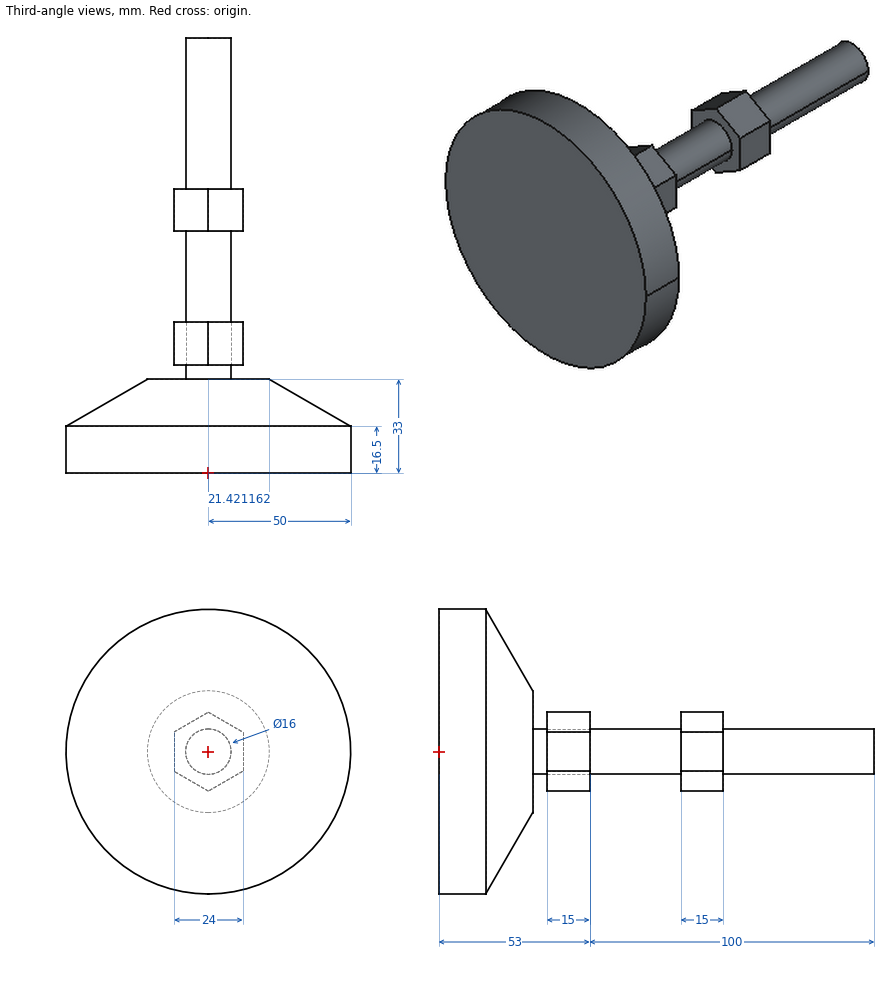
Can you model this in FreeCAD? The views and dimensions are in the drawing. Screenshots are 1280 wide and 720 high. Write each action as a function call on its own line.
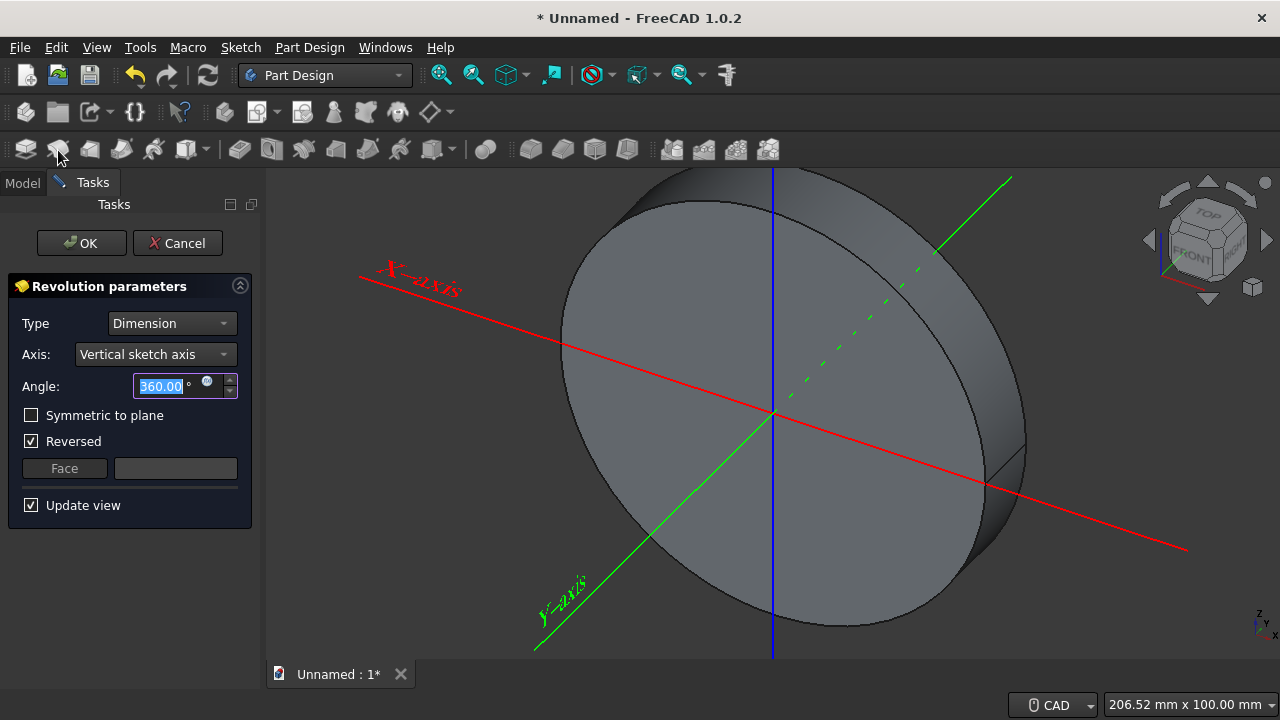
click(82, 243)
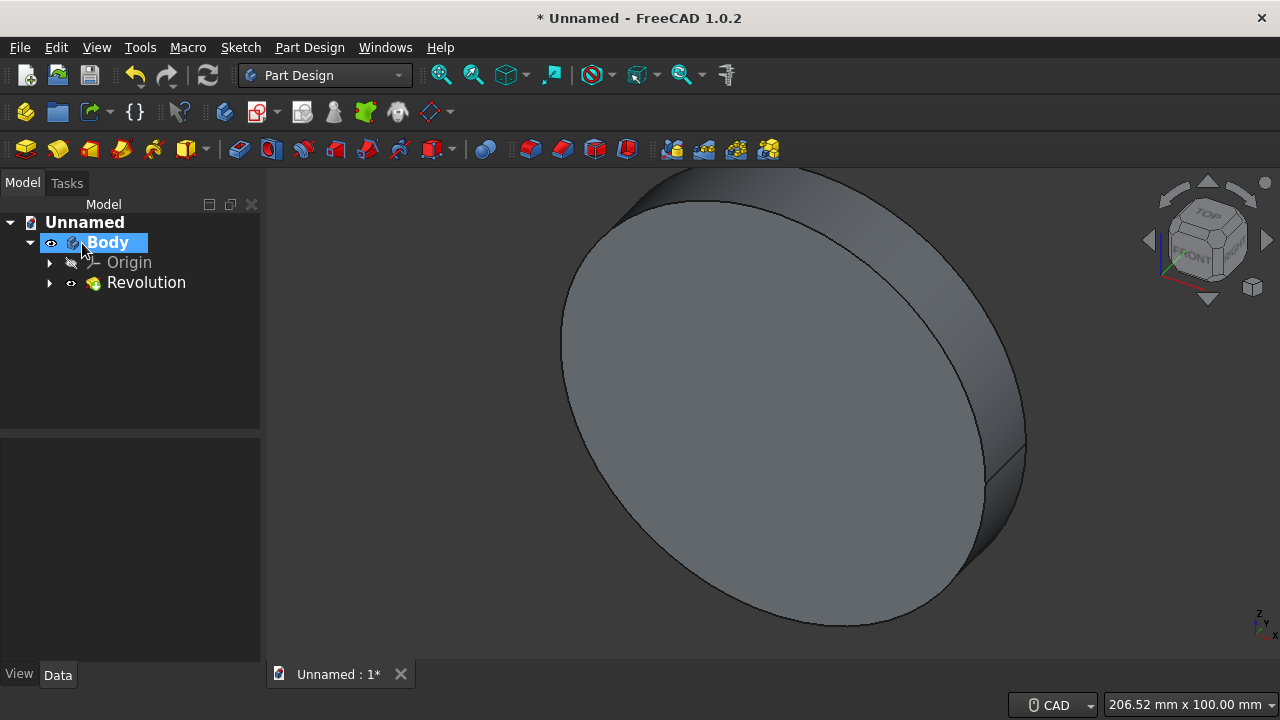
click(442, 76)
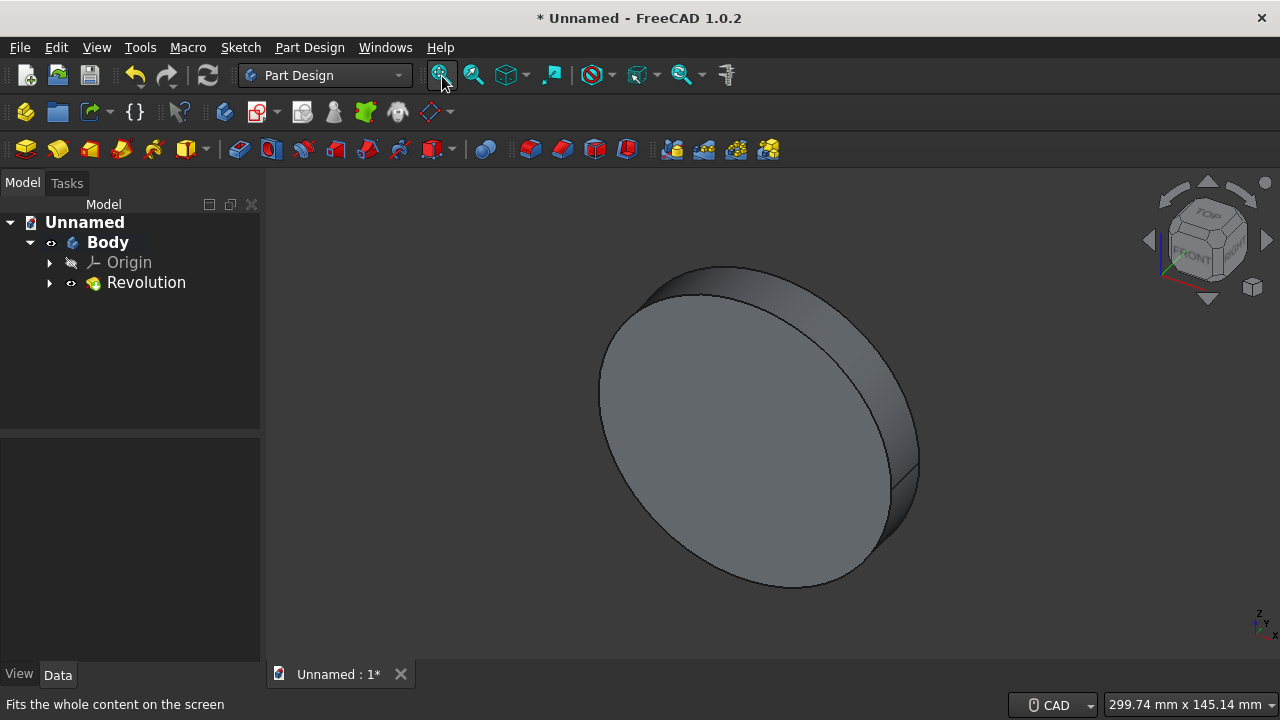
click(50, 263)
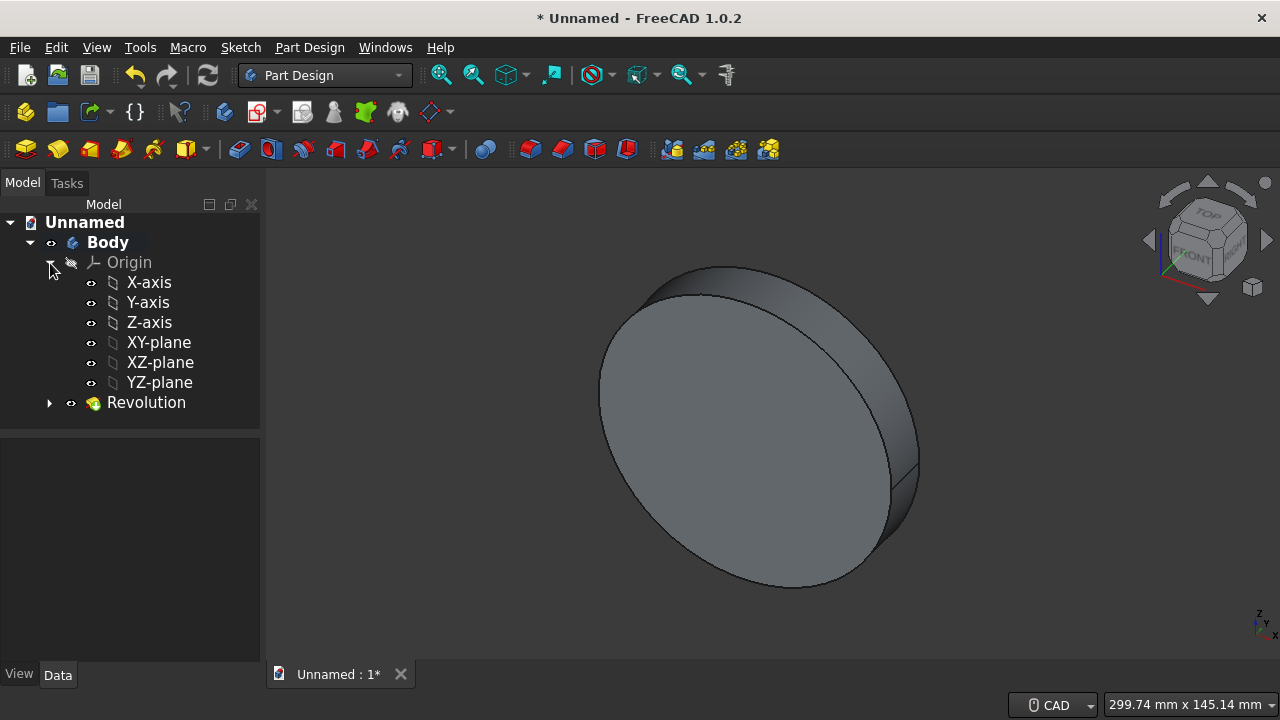
click(136, 363)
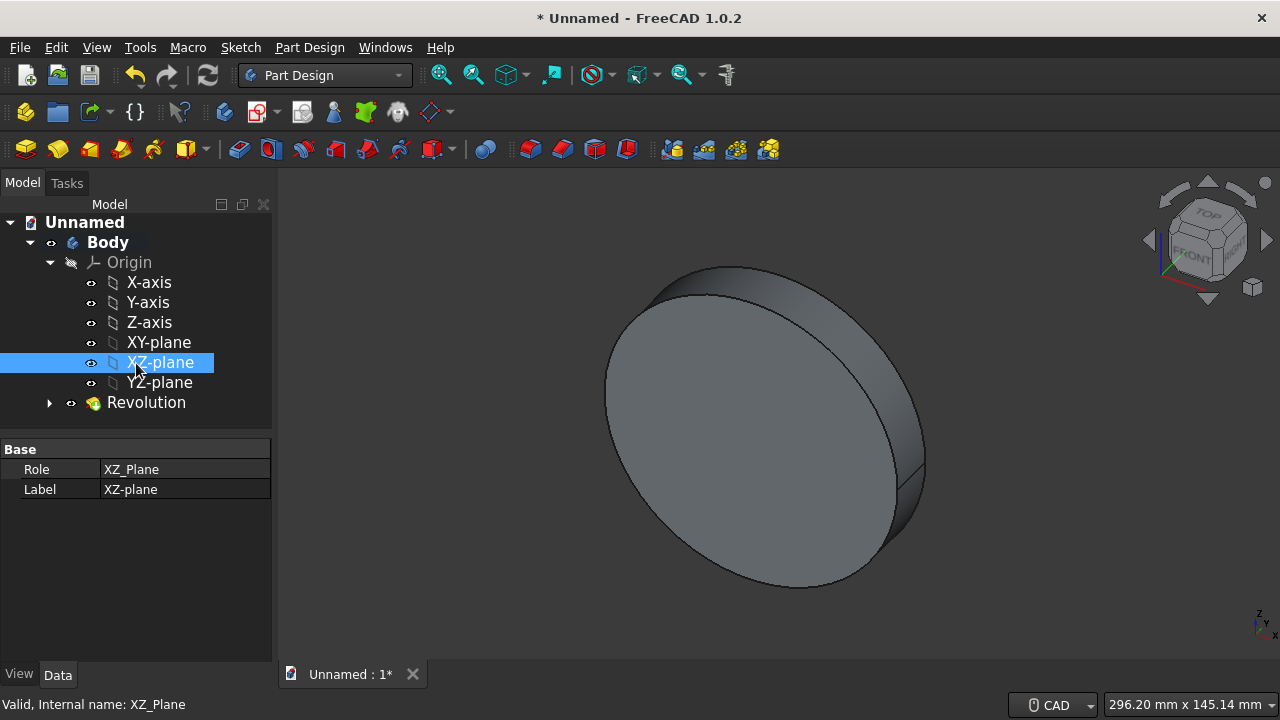
click(430, 112)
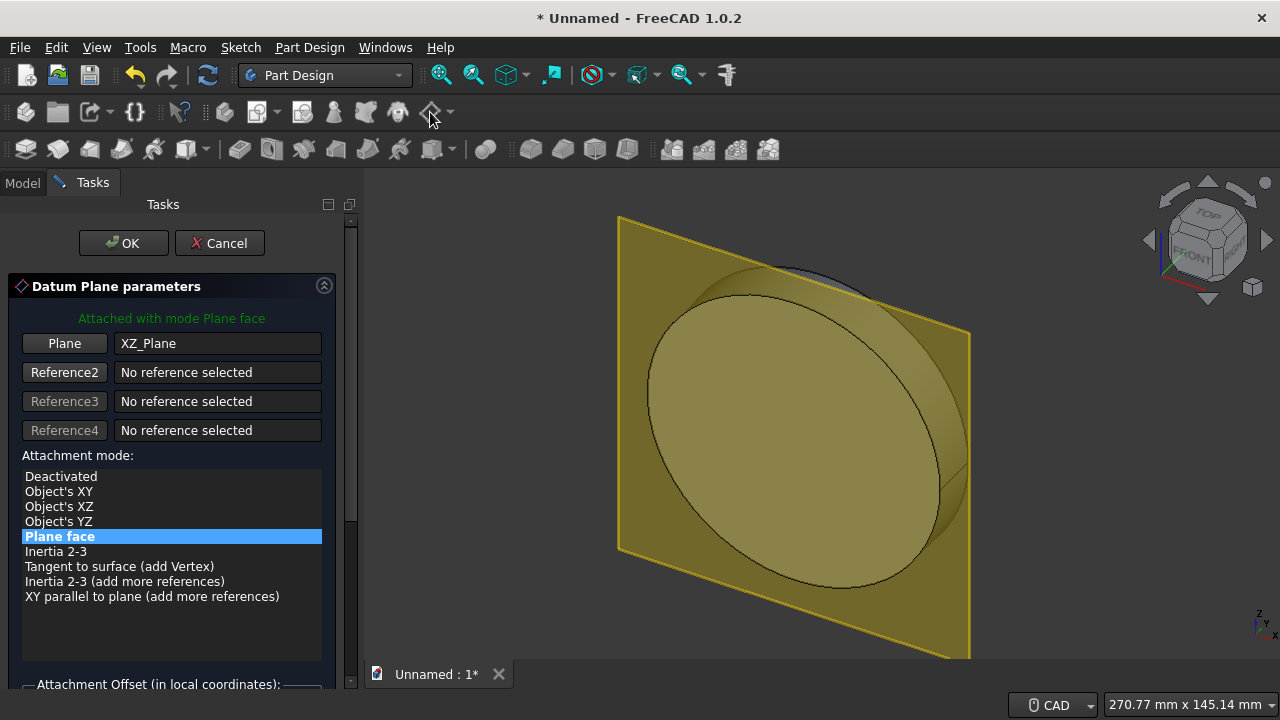
scroll(351, 451, down, 3)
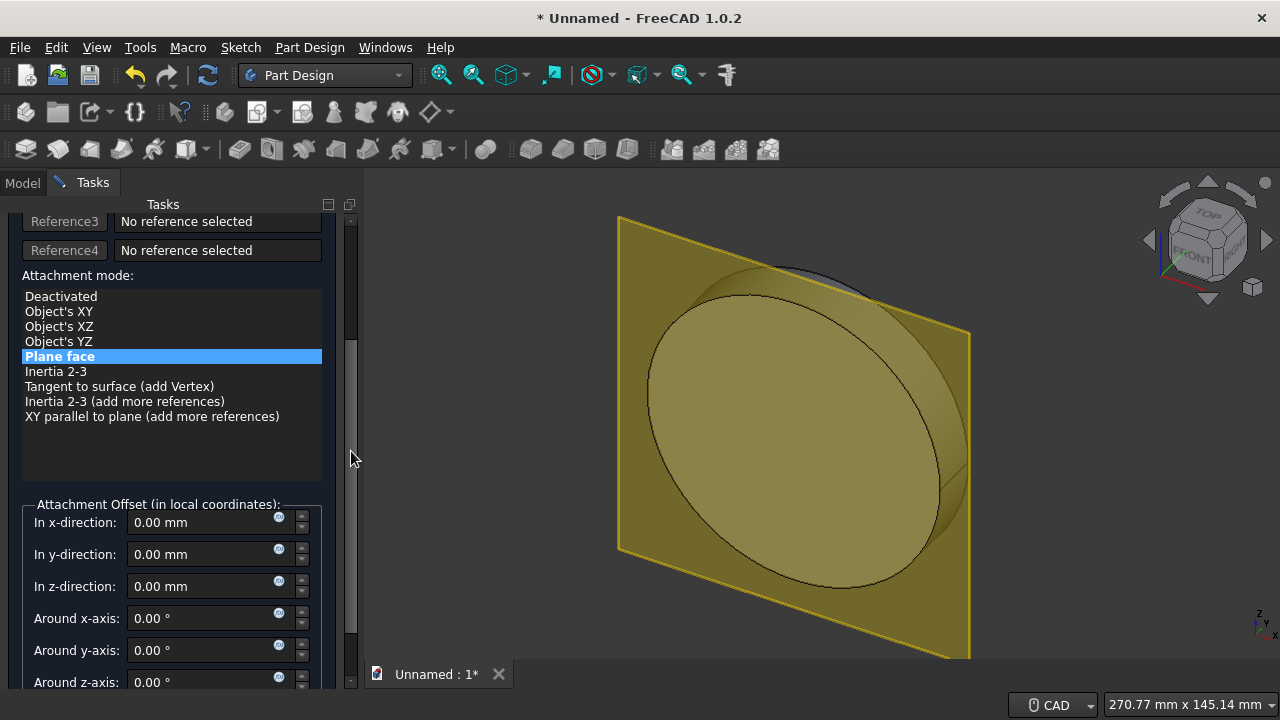
triple_click(210, 586)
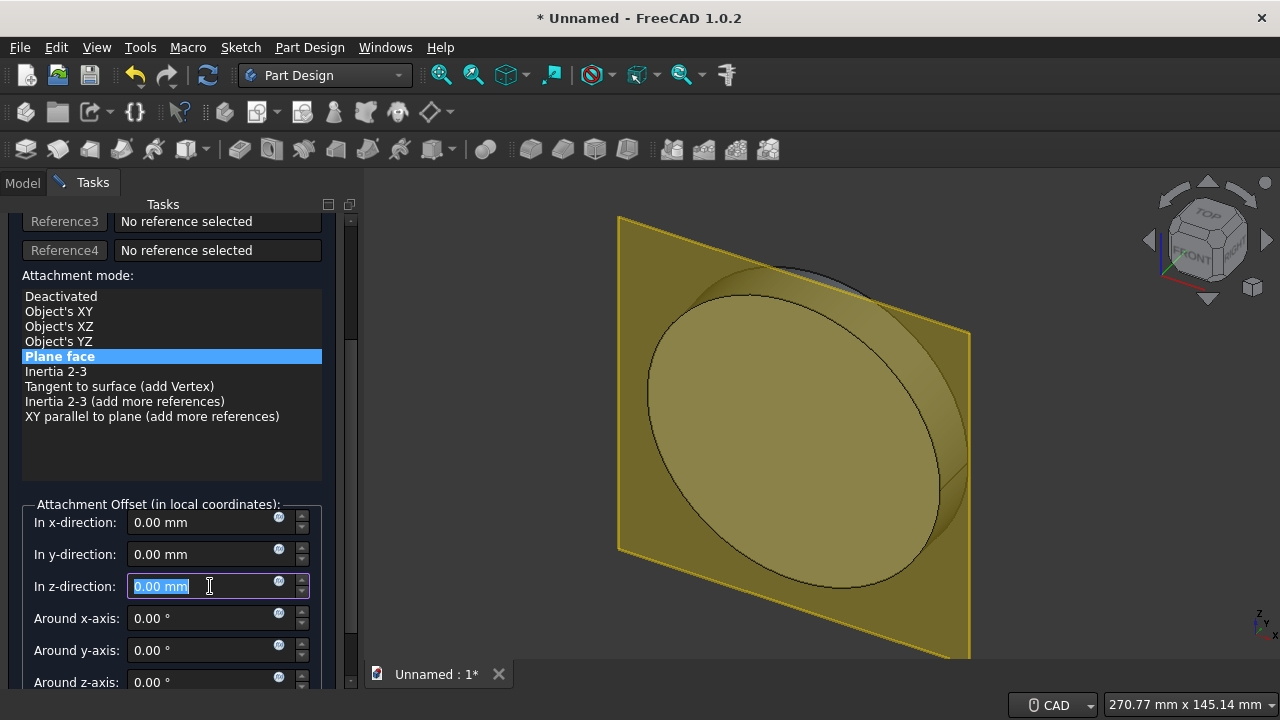
text(-53)
key(Tab)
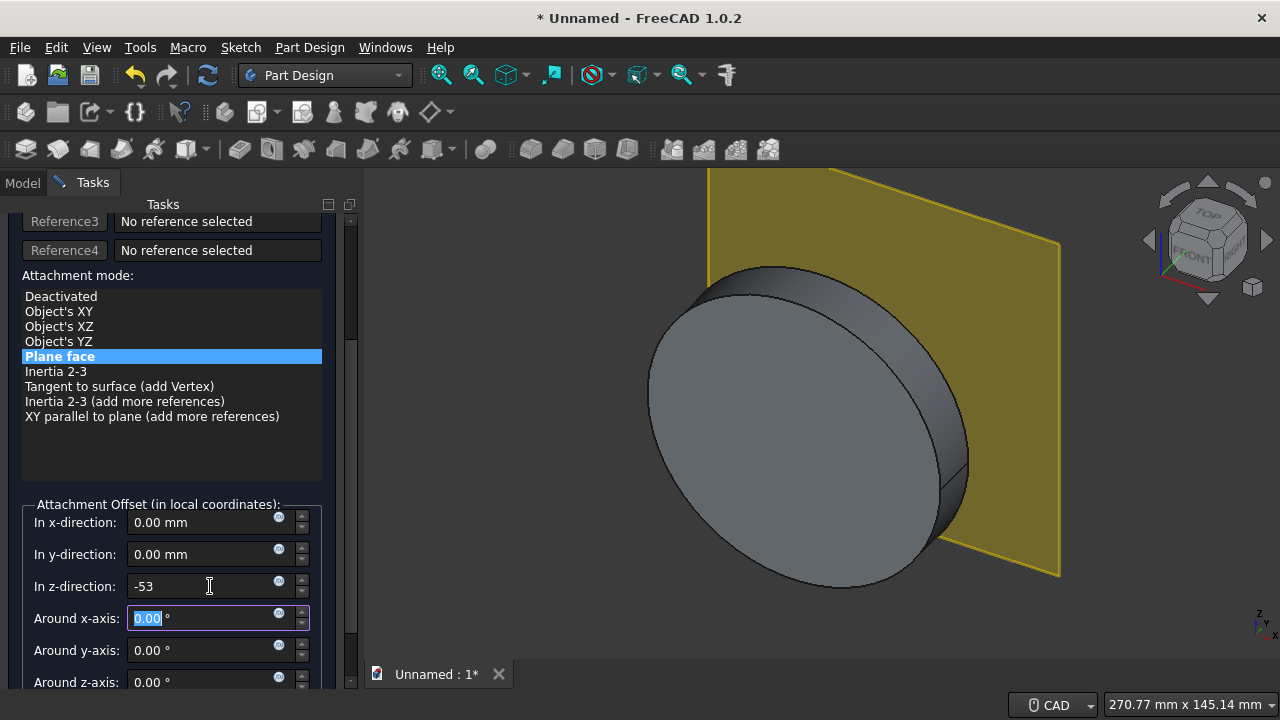
scroll(351, 451, up, 4)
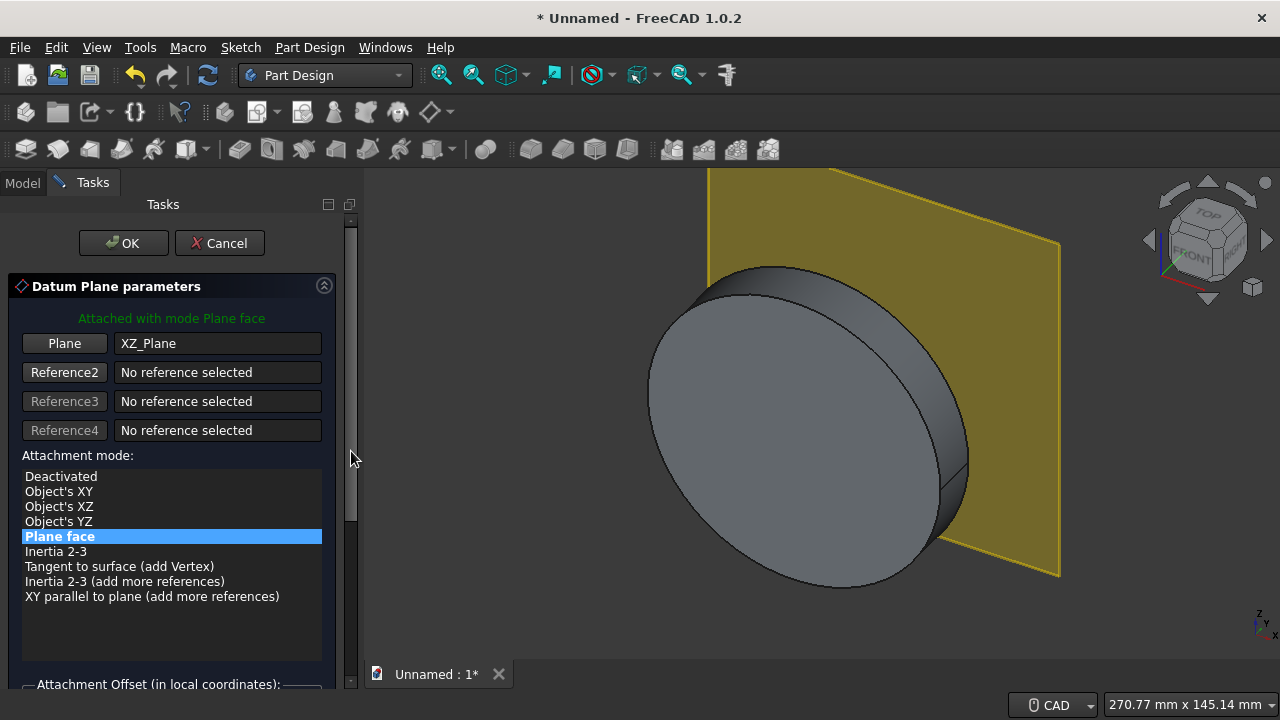
click(124, 243)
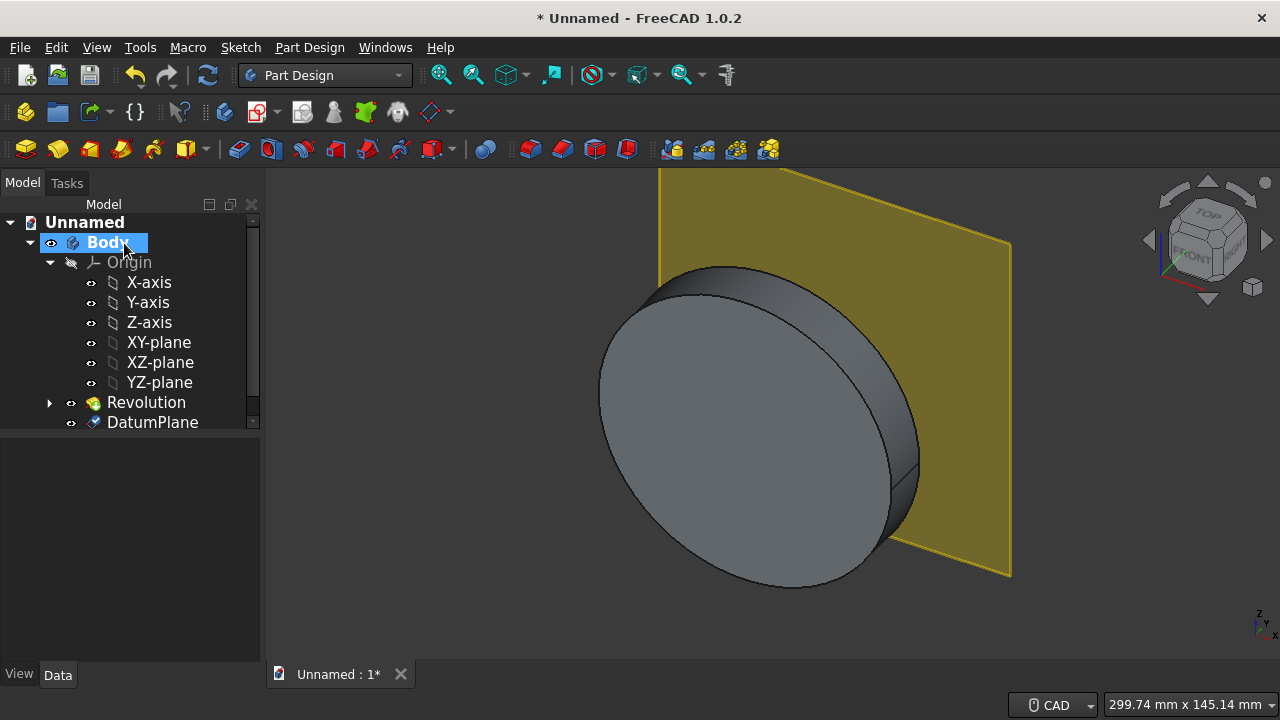
click(116, 423)